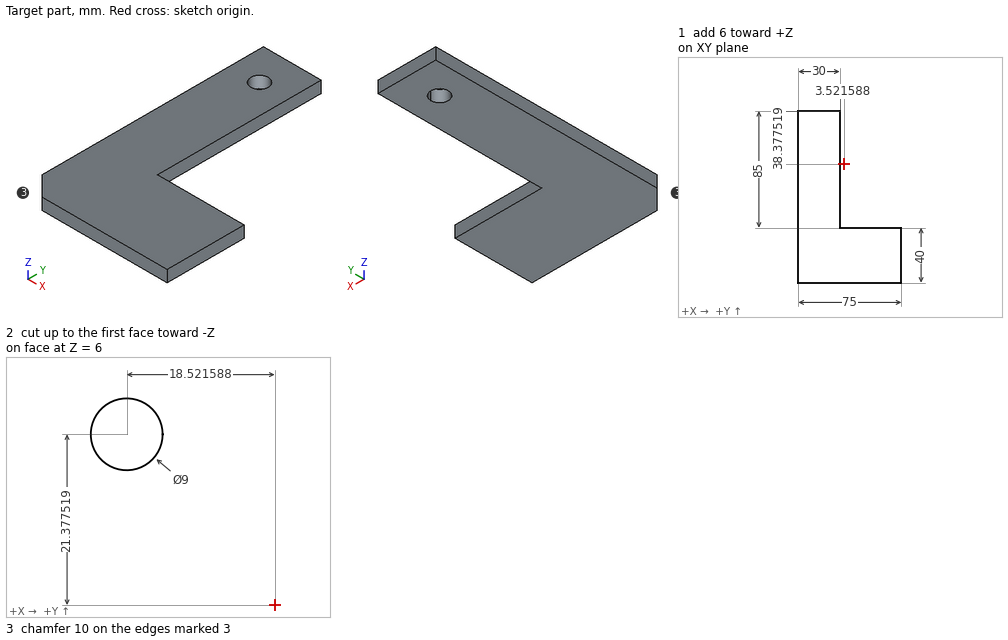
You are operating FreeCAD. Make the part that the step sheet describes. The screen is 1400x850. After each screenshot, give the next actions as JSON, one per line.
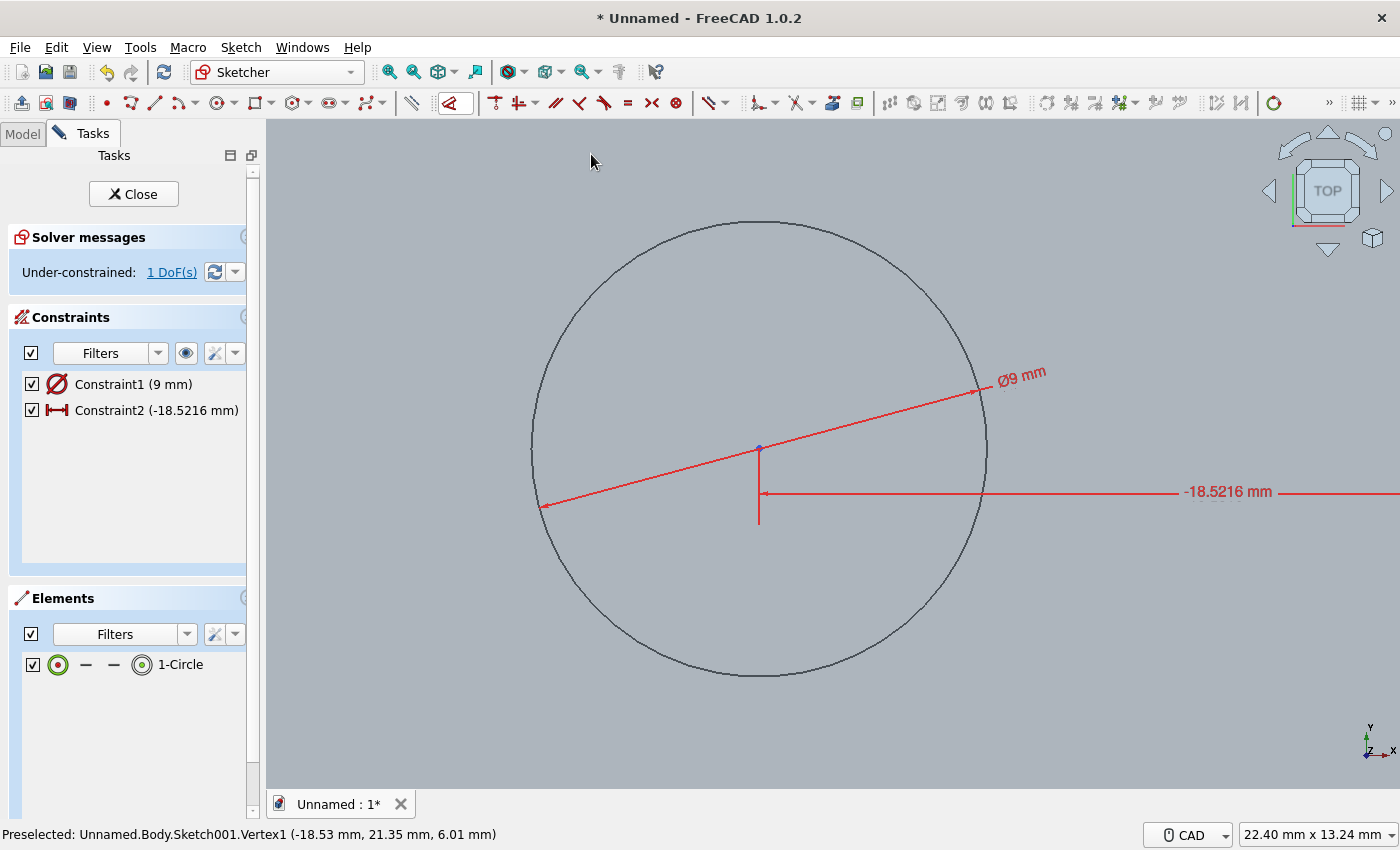
{"action": "left_click", "coordinate": [759, 449]}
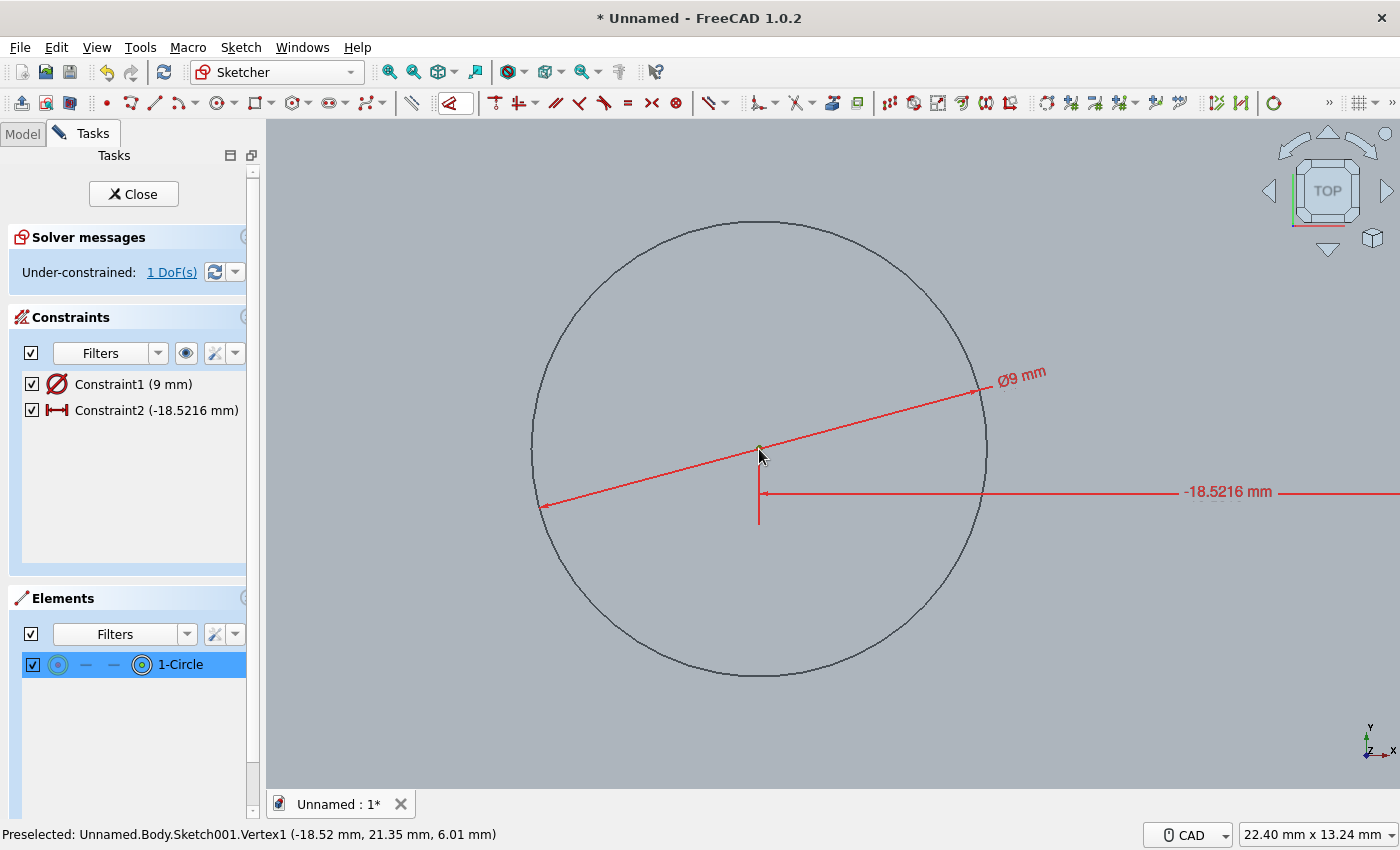
{"action": "key", "text": "i"}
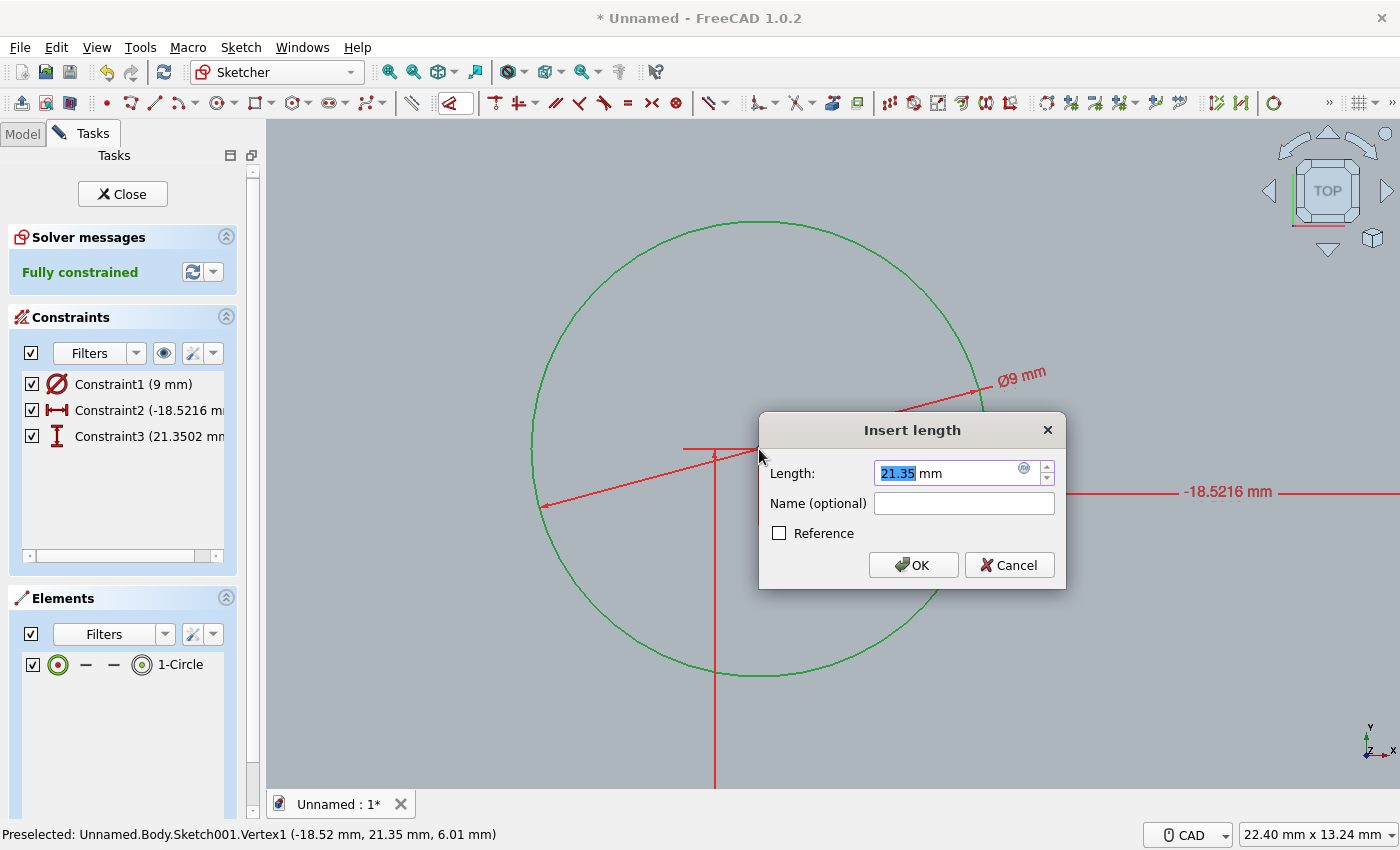
{"action": "type", "text": "21.377519"}
{"action": "key", "text": "Return"}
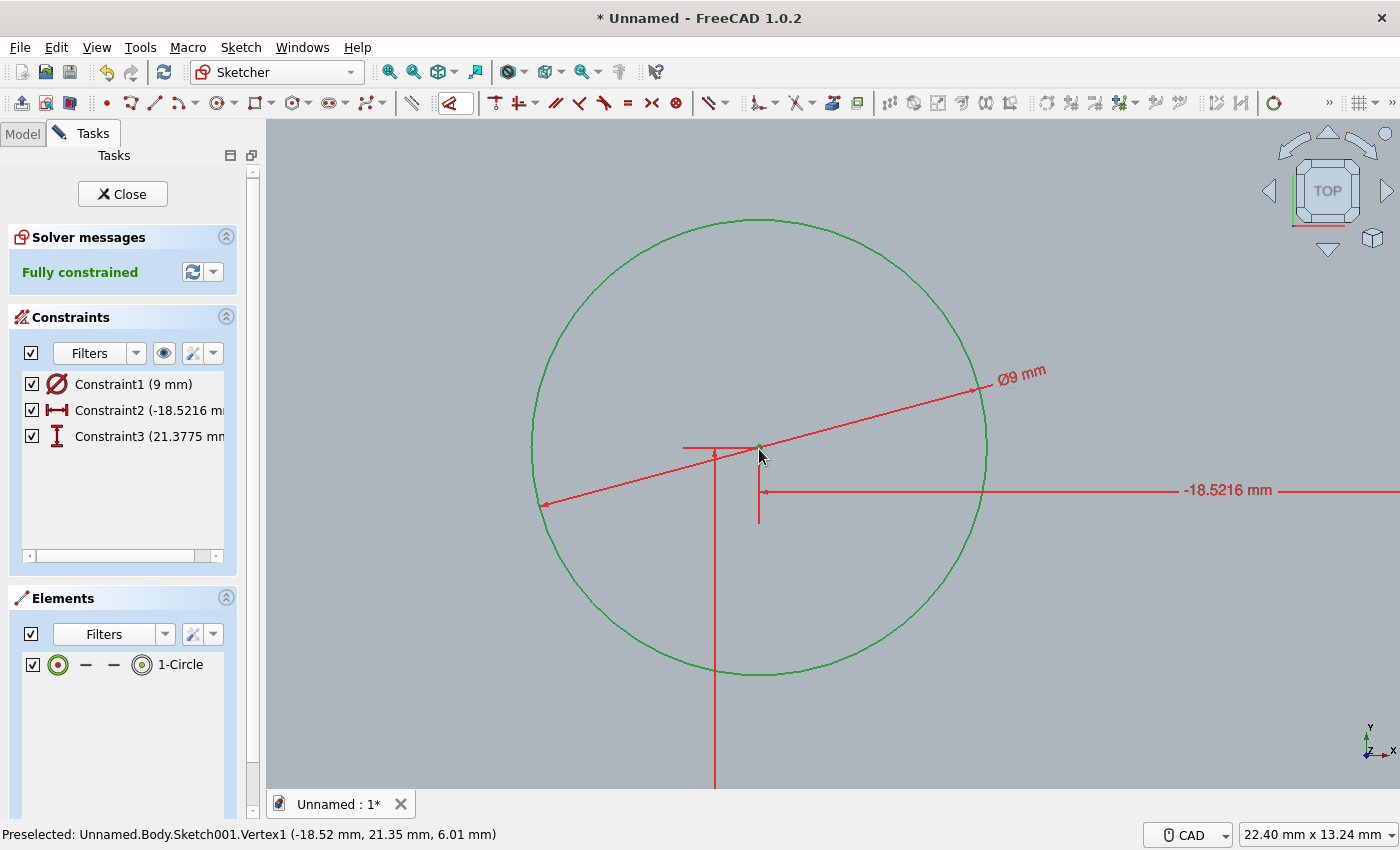
{"action": "left_click", "coordinate": [123, 194]}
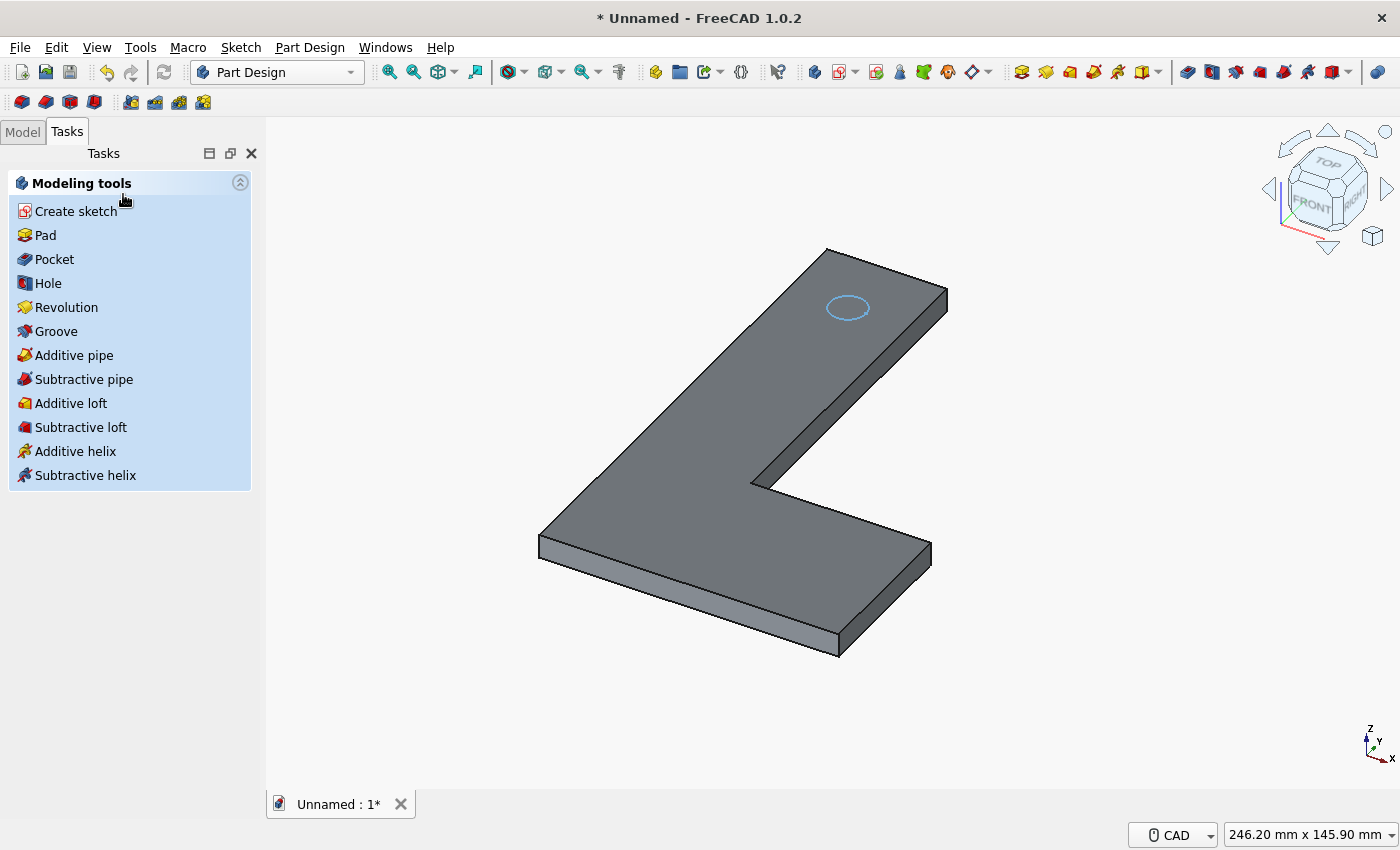
{"action": "left_click", "coordinate": [1188, 72]}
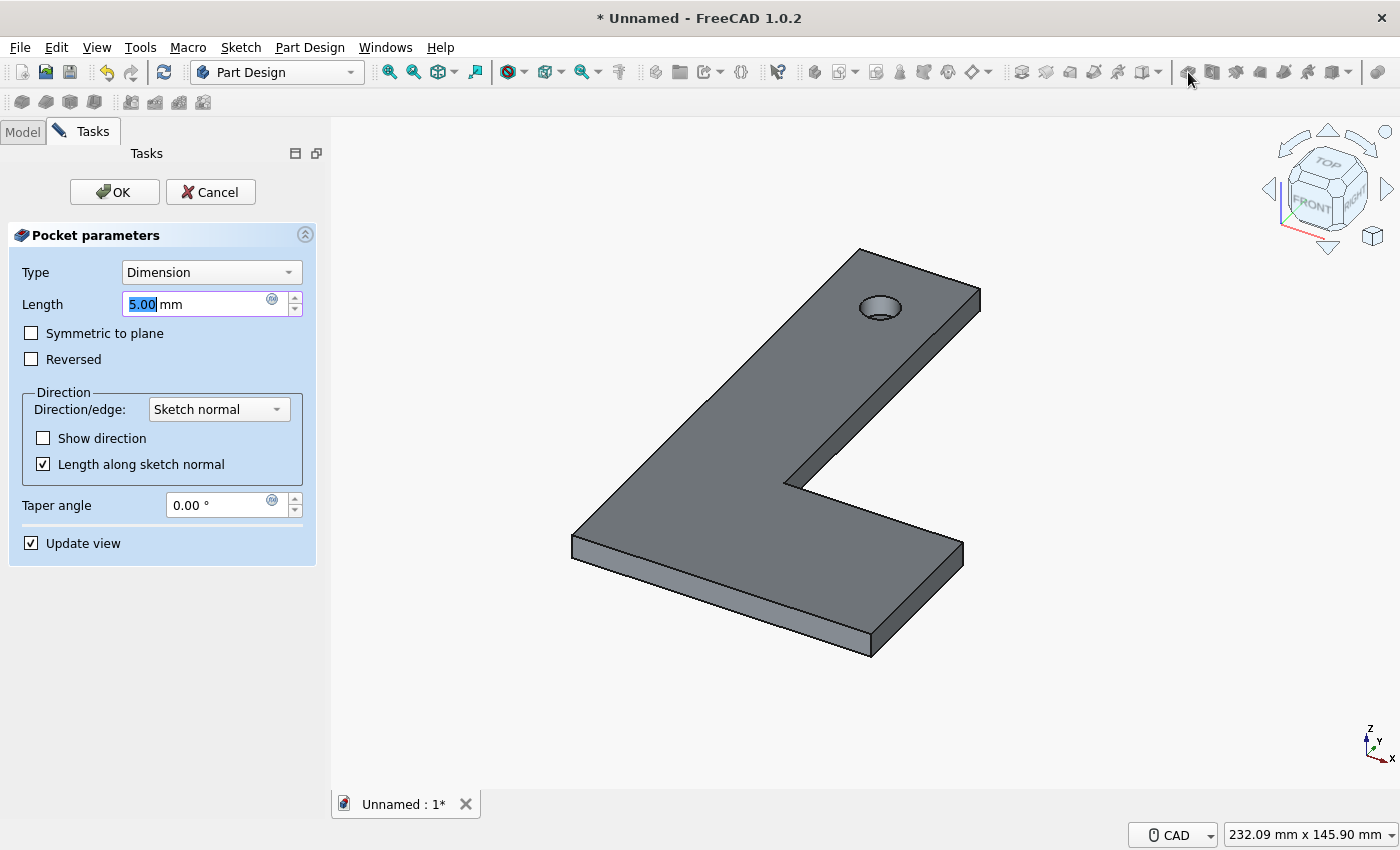
{"action": "left_click", "coordinate": [212, 272]}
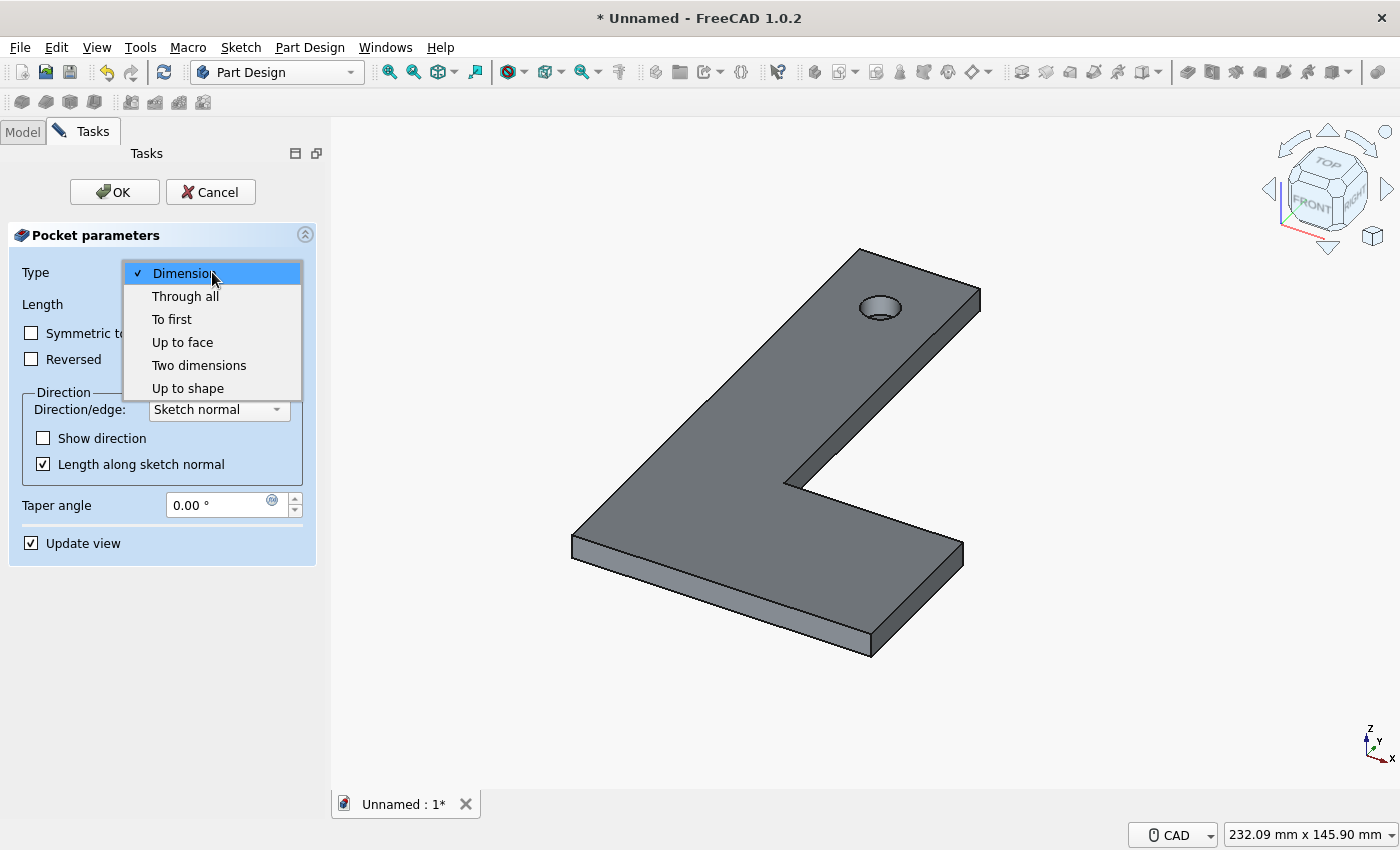
{"action": "left_click", "coordinate": [212, 320]}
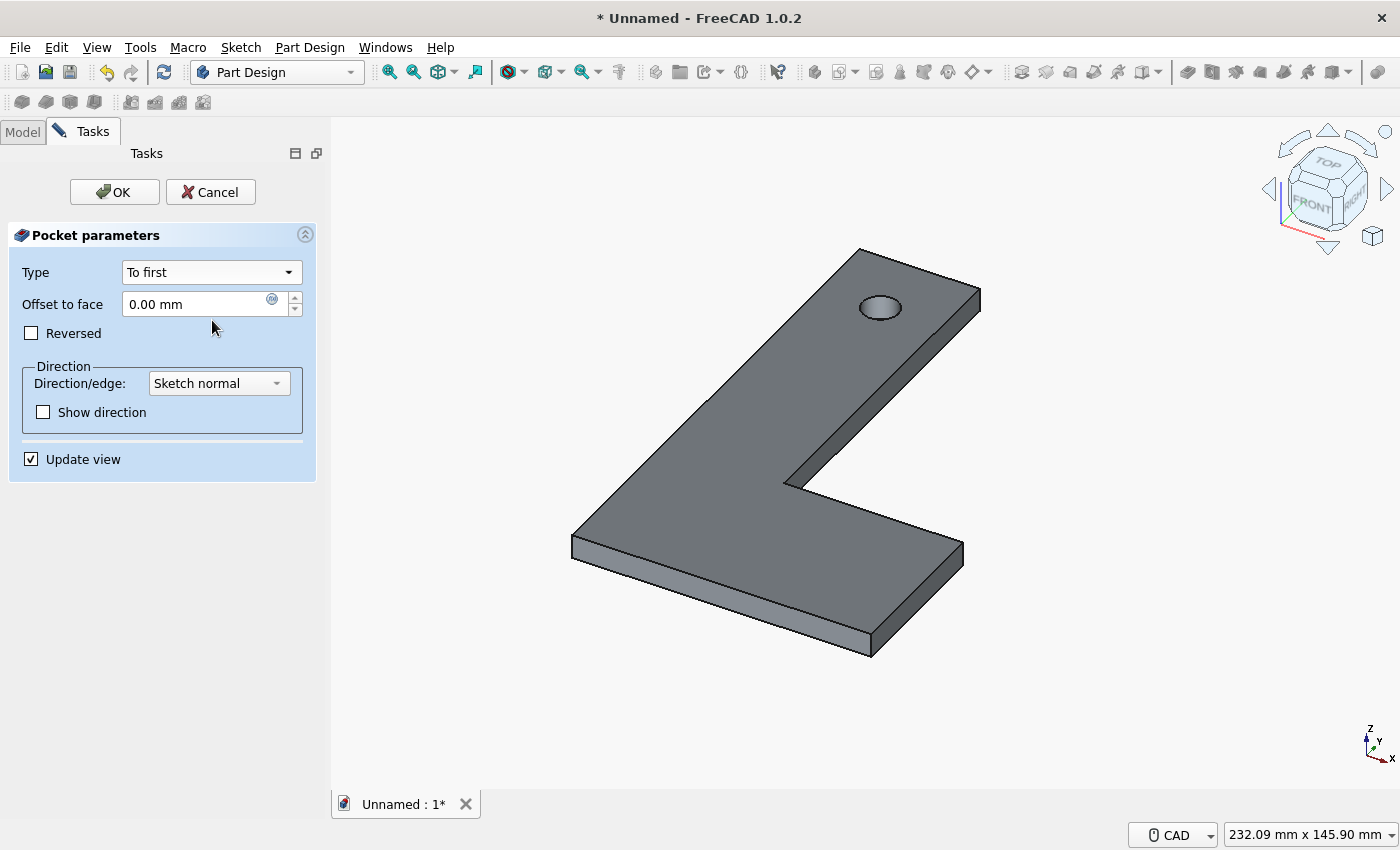
{"action": "left_click", "coordinate": [115, 192]}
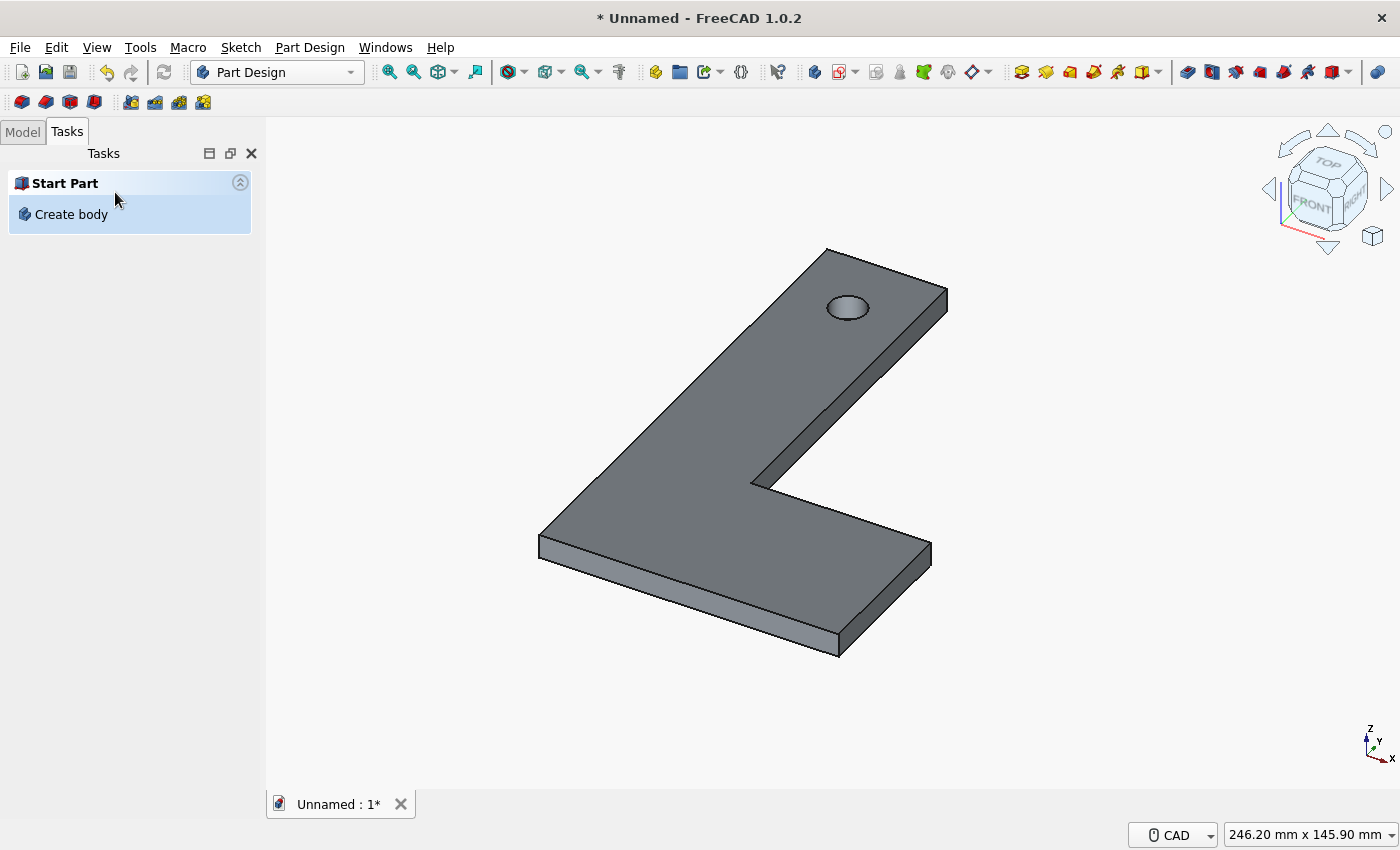
{"action": "key", "text": "0"}